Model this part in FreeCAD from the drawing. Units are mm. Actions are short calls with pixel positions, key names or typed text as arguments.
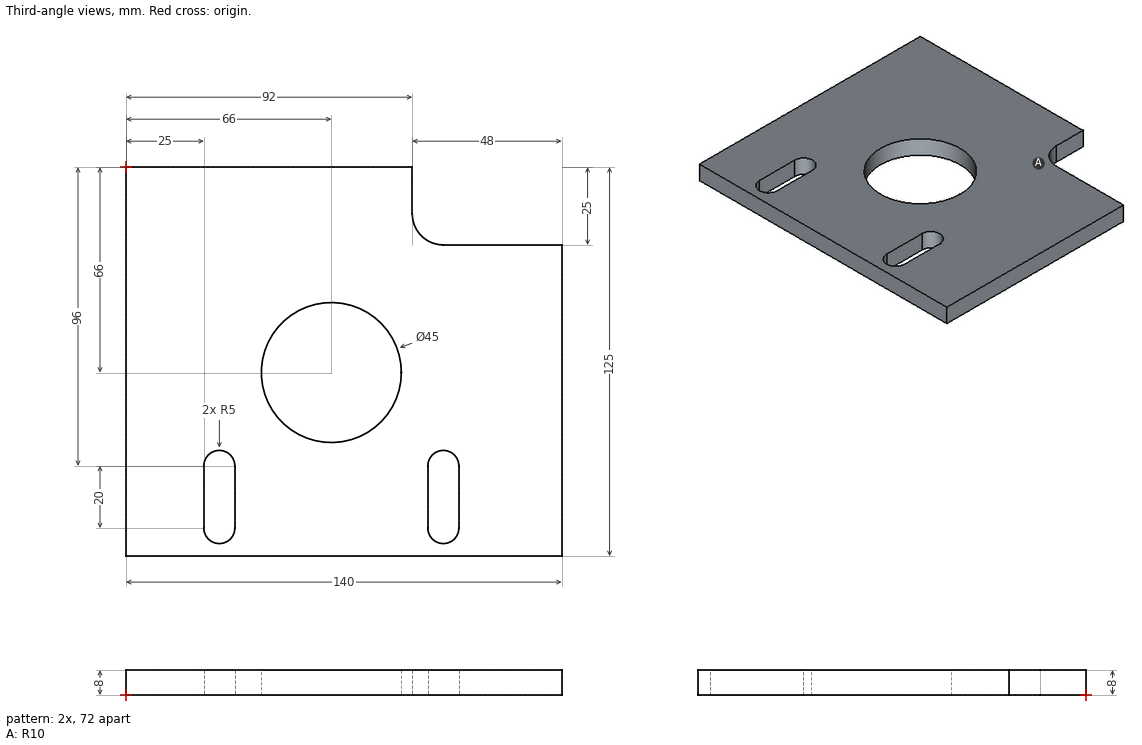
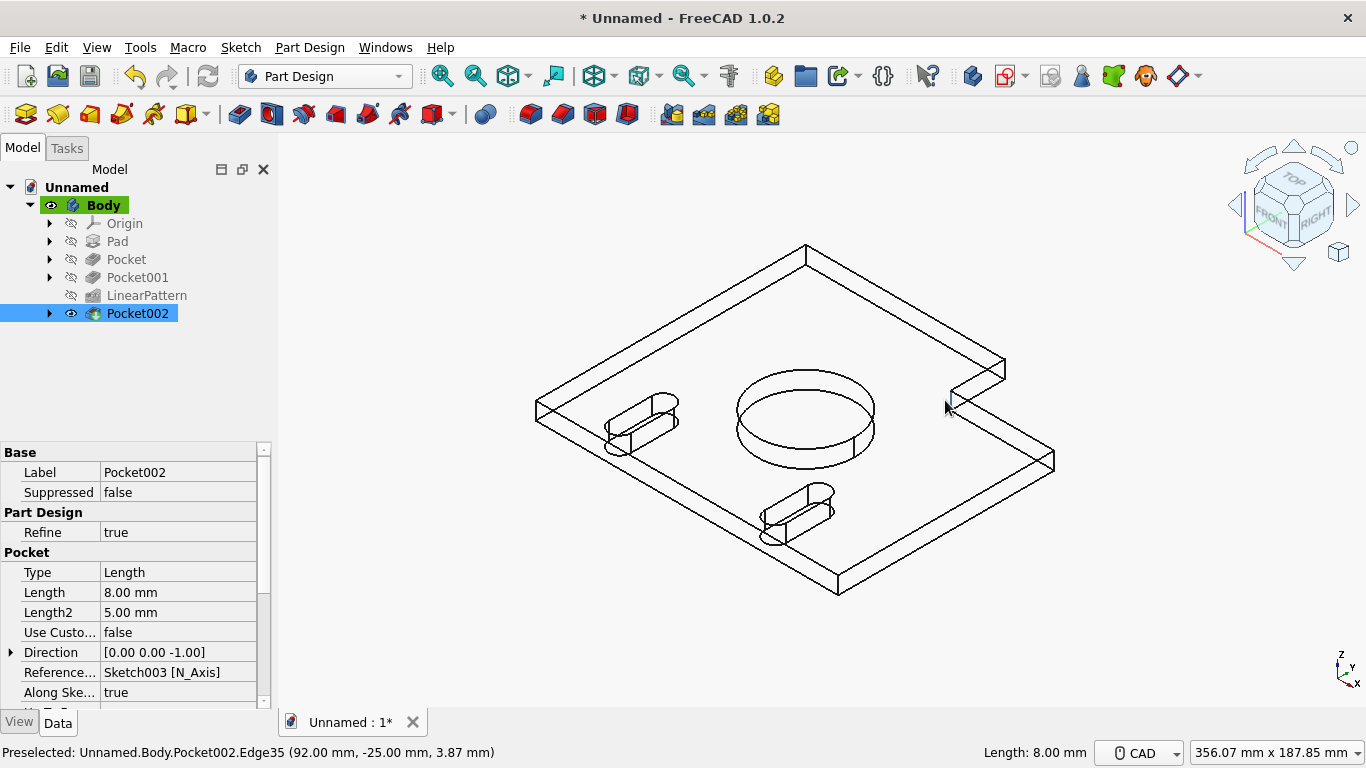
key(v)
key(1)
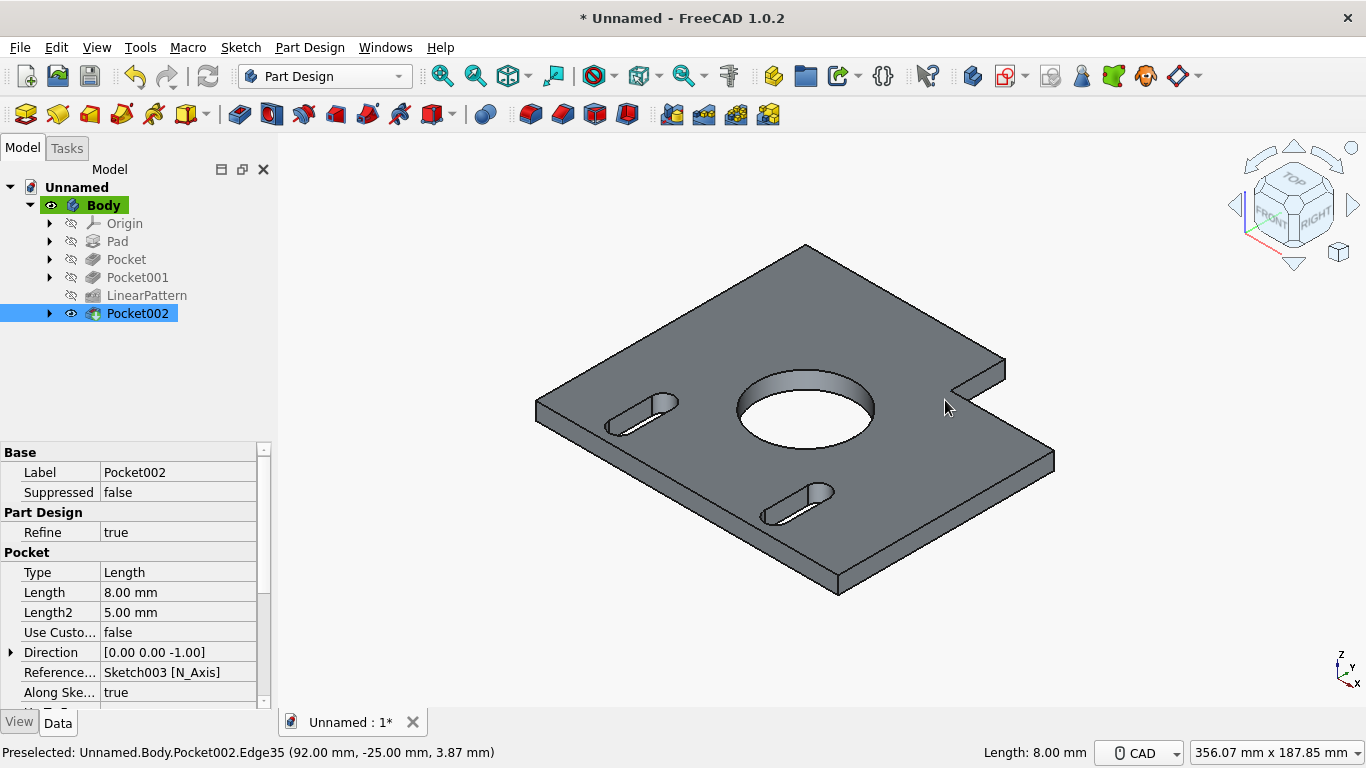
click(532, 114)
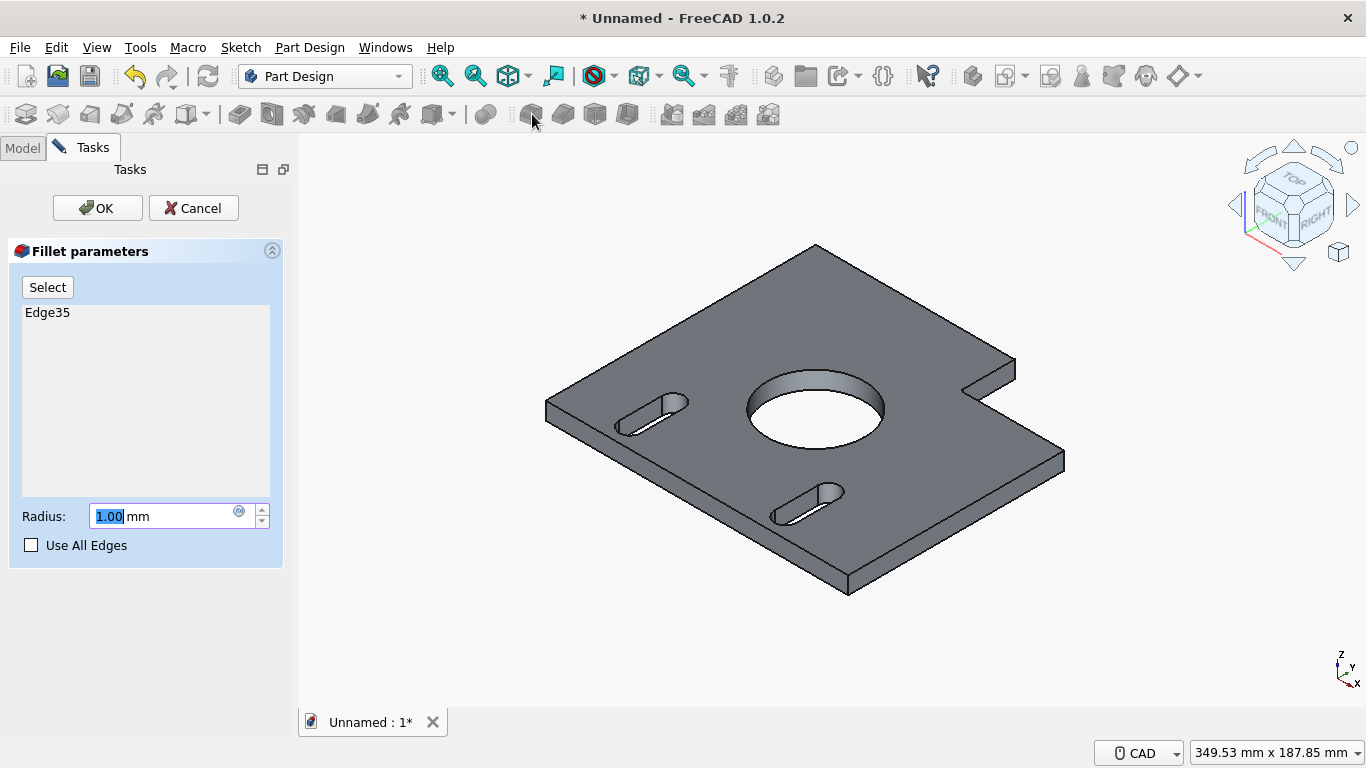
text(10)
key(Tab)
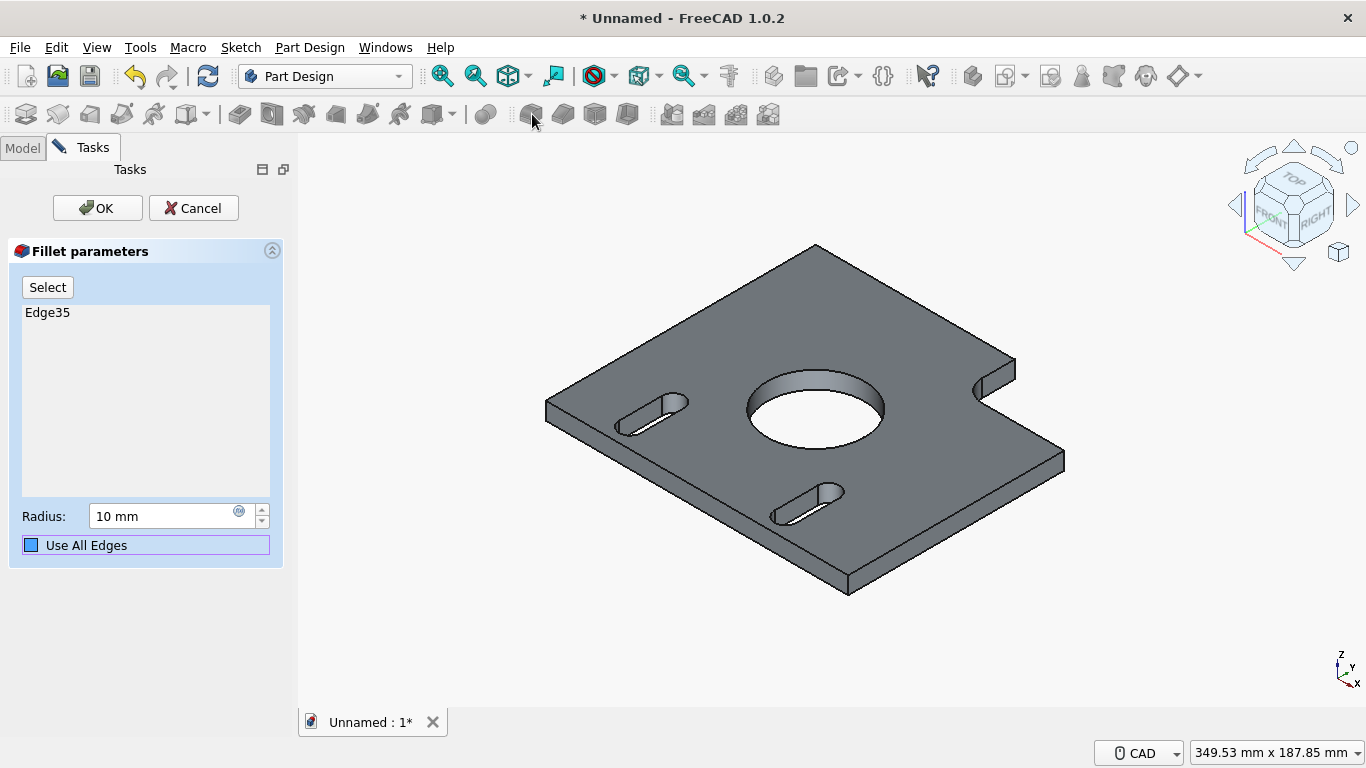
click(98, 208)